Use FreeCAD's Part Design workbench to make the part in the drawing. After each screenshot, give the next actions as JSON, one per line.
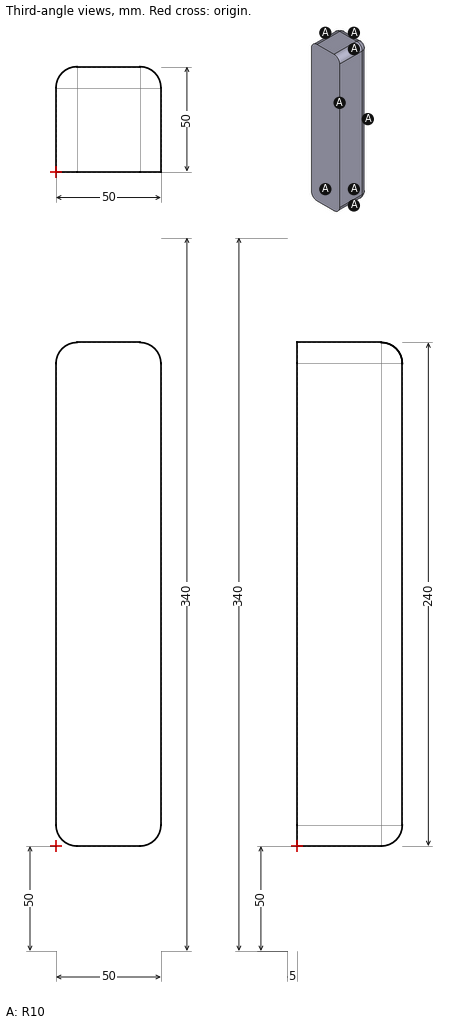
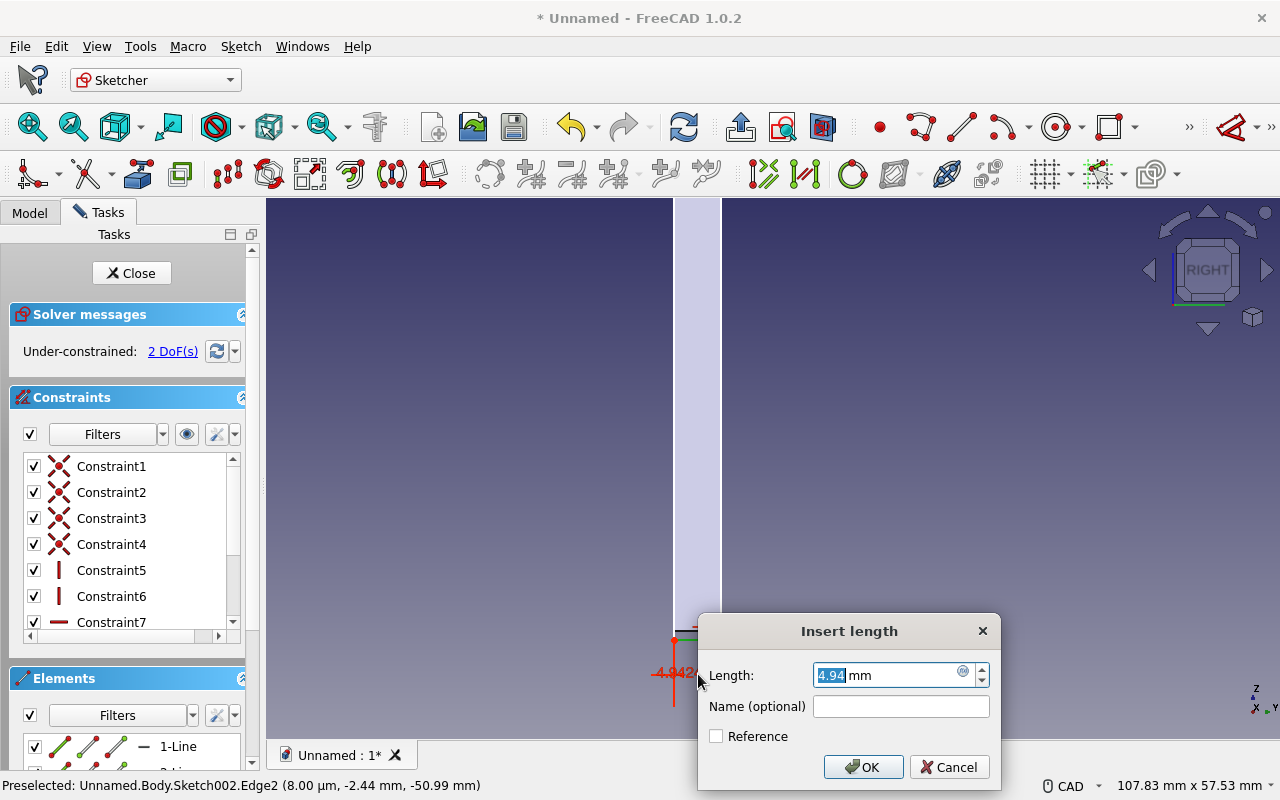
{"action": "type", "text": "5"}
{"action": "key", "text": "Return"}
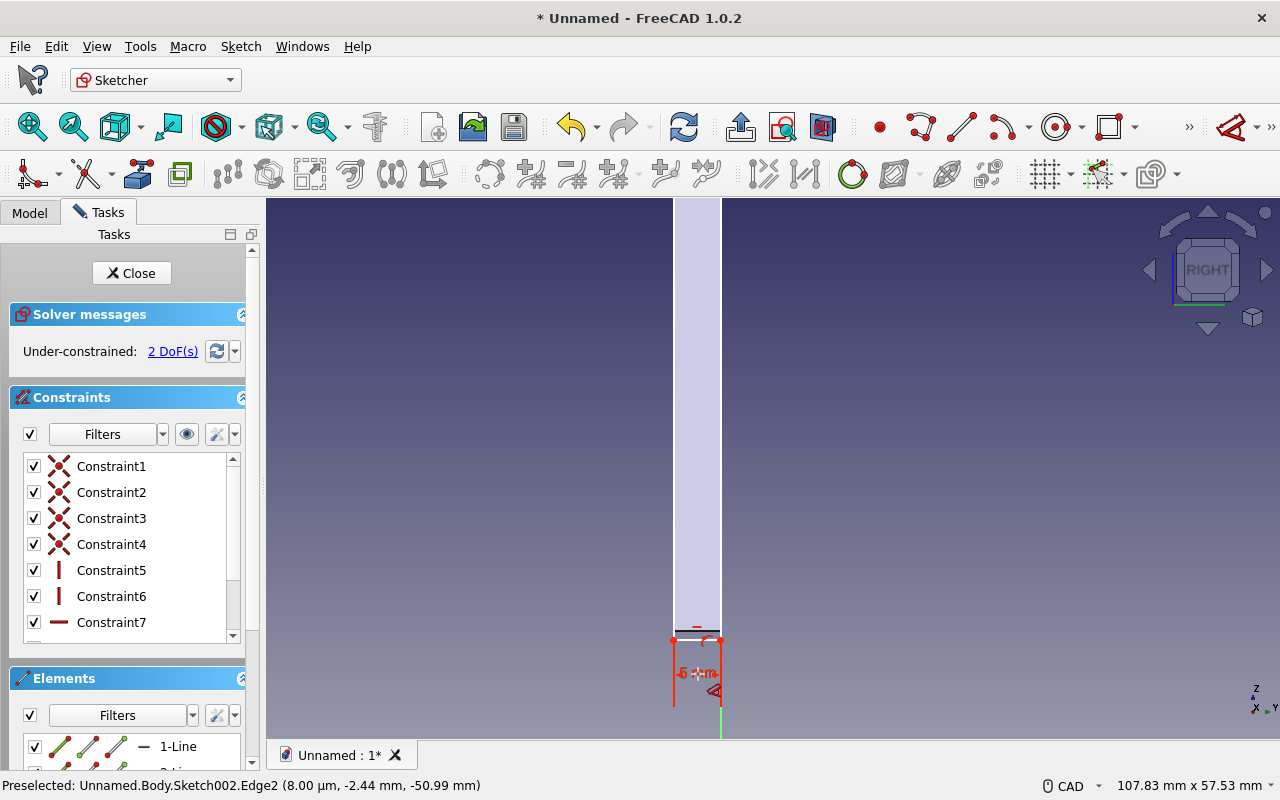
{"action": "scroll", "coordinate": [705, 647], "scroll_direction": "down", "scroll_amount": 11}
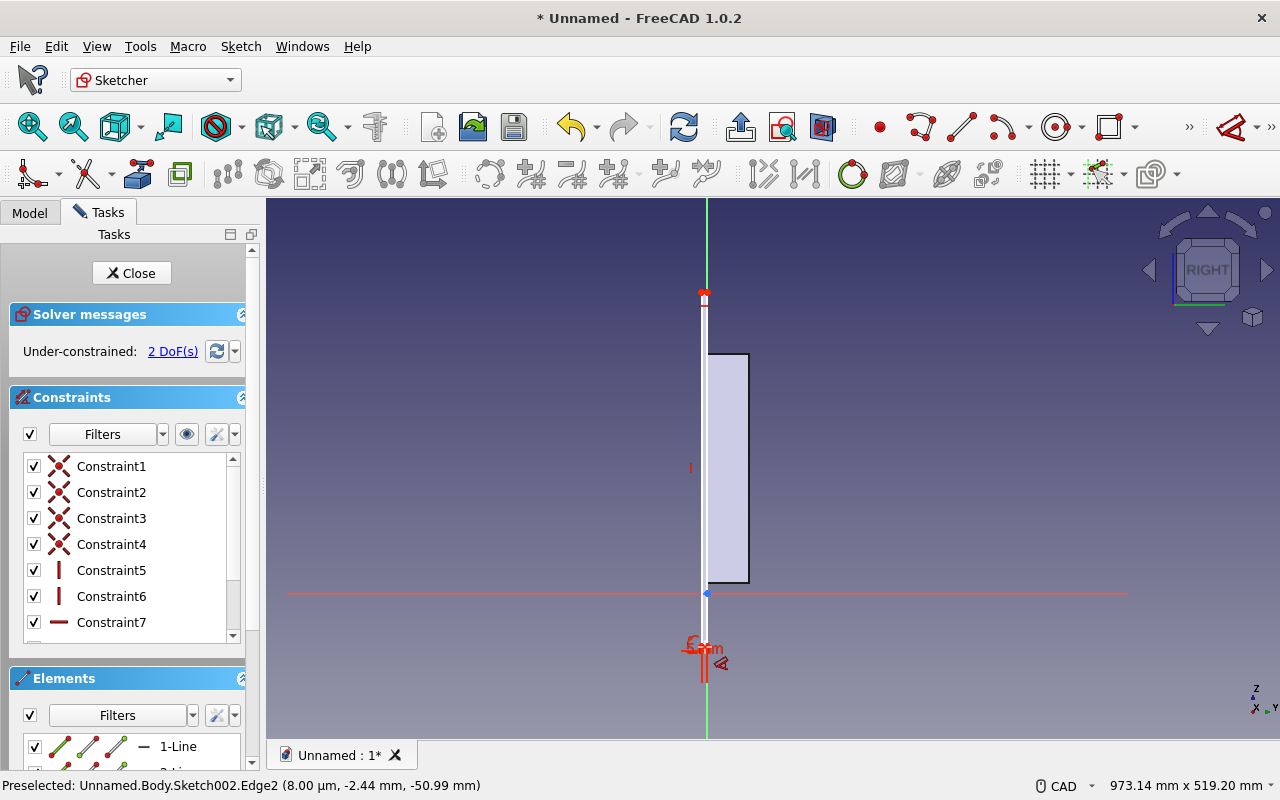
{"action": "scroll", "coordinate": [702, 399], "scroll_direction": "up", "scroll_amount": 5}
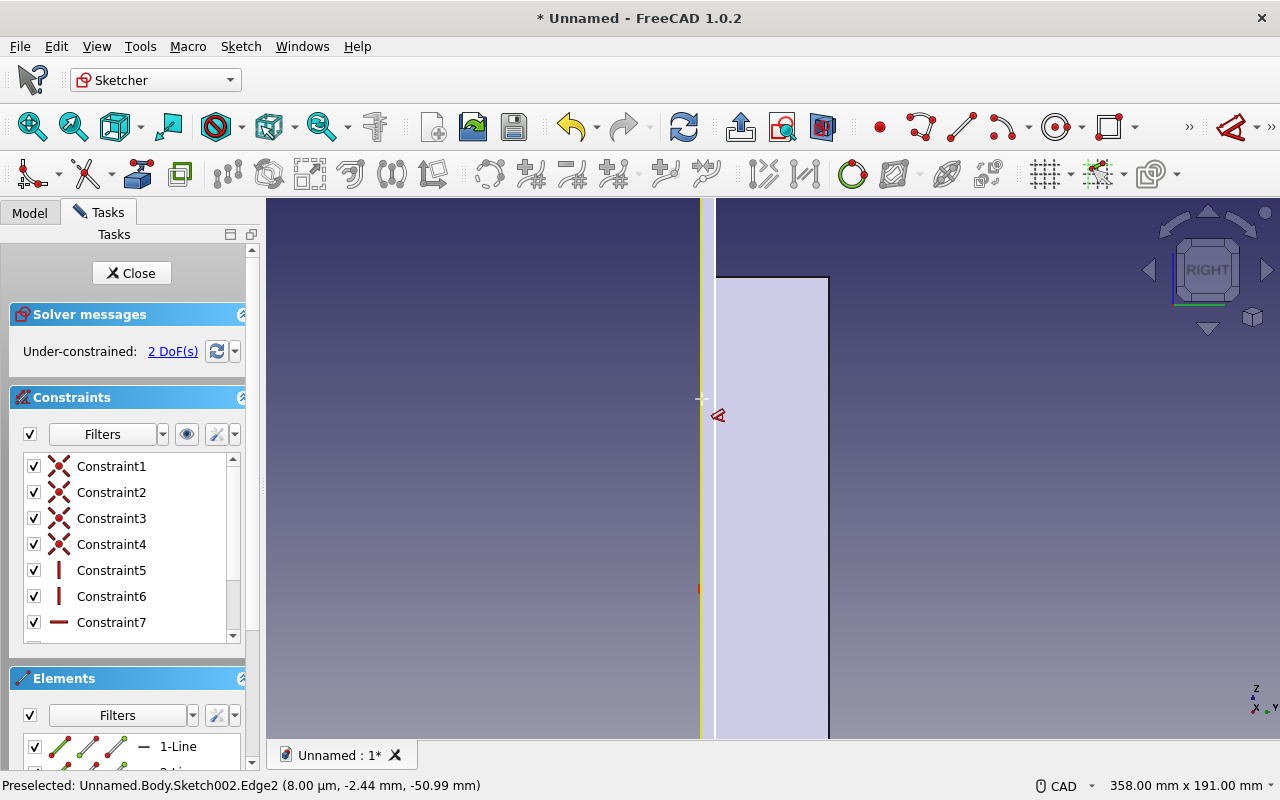
{"action": "left_click", "coordinate": [701, 397]}
{"action": "left_click", "coordinate": [667, 468]}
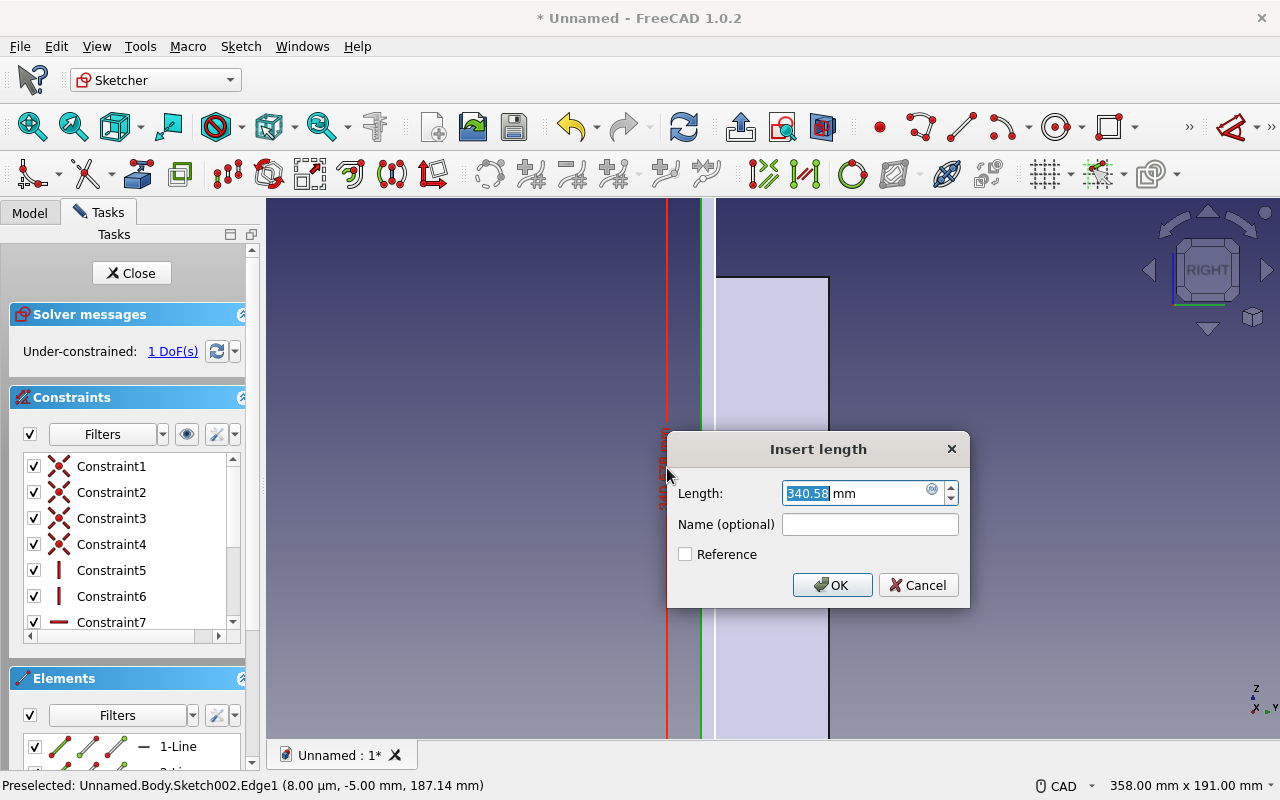
{"action": "type", "text": "340"}
{"action": "key", "text": "Return"}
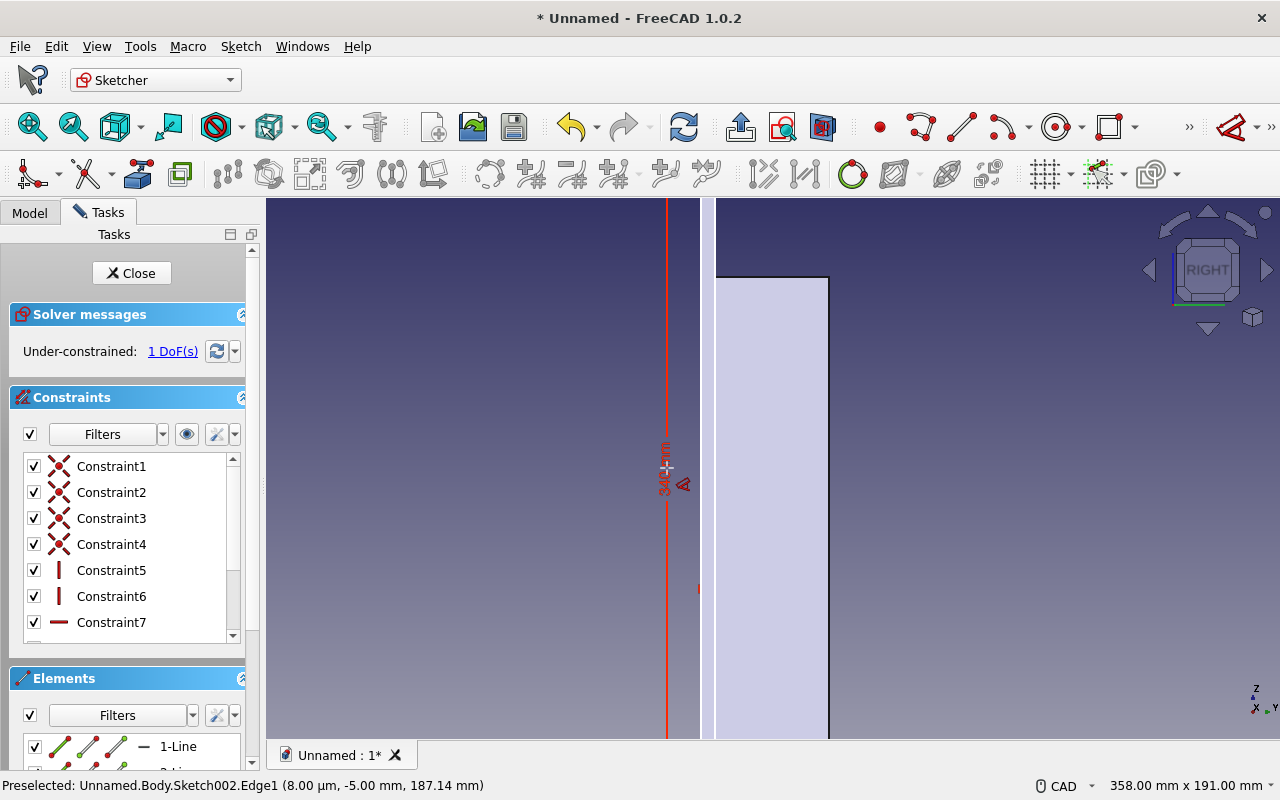
{"action": "scroll", "coordinate": [702, 399], "scroll_direction": "down", "scroll_amount": 5}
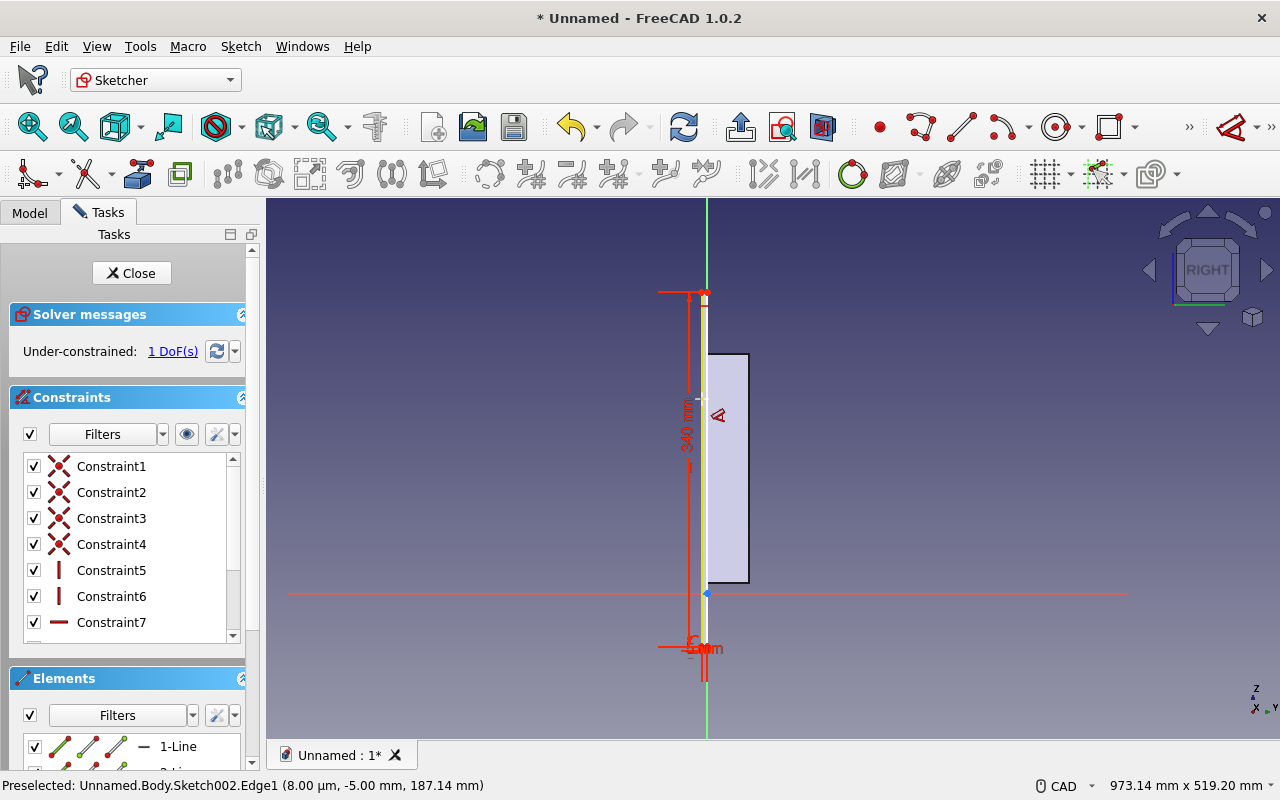
{"action": "scroll", "coordinate": [702, 647], "scroll_direction": "up", "scroll_amount": 5}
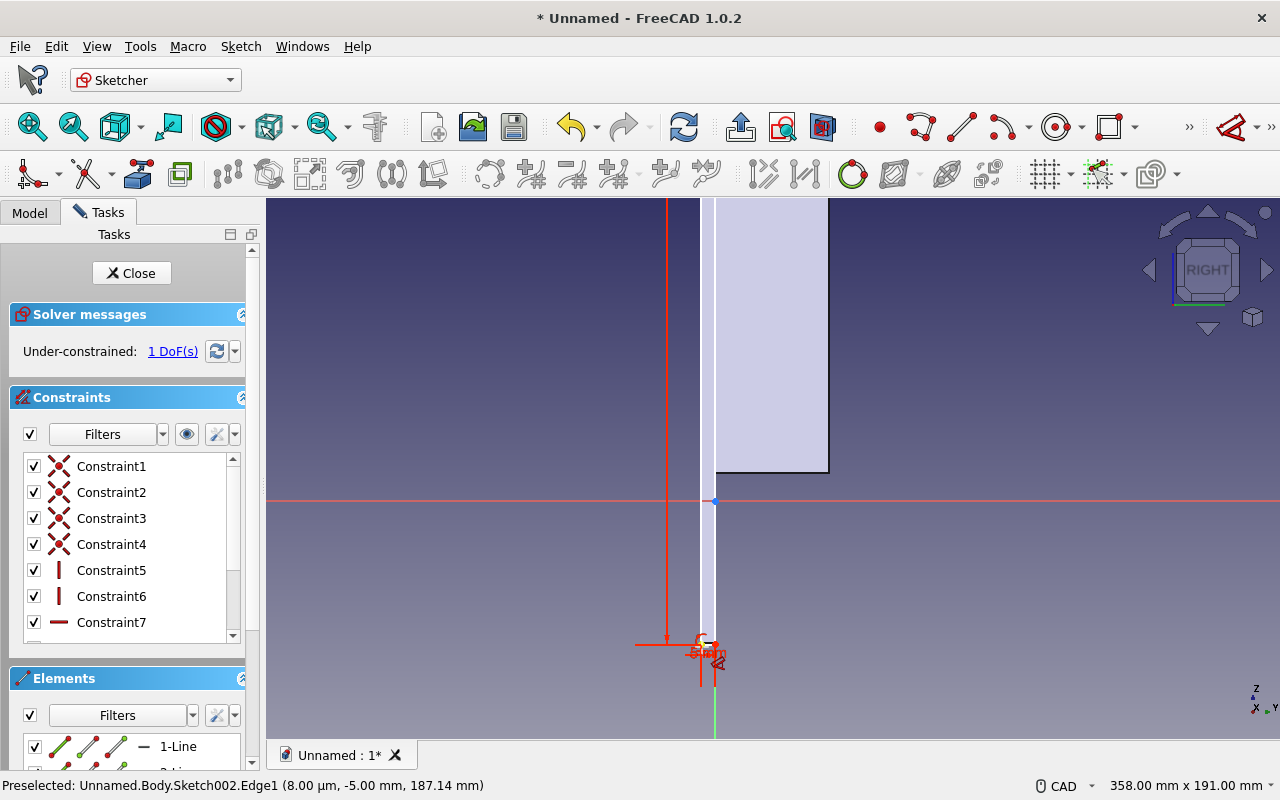
{"action": "left_click", "coordinate": [701, 645]}
{"action": "left_click", "coordinate": [667, 573]}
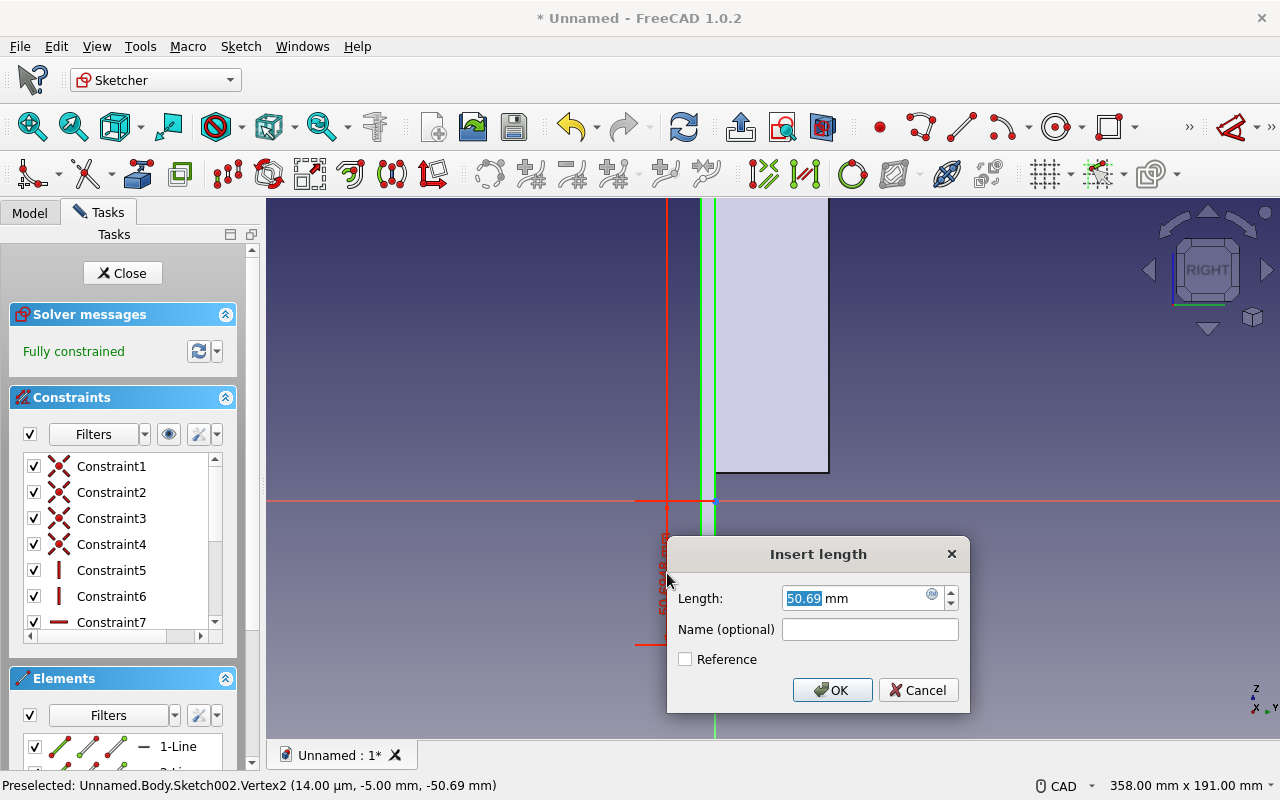
{"action": "type", "text": "50"}
{"action": "key", "text": "Return"}
{"action": "key", "text": "Escape"}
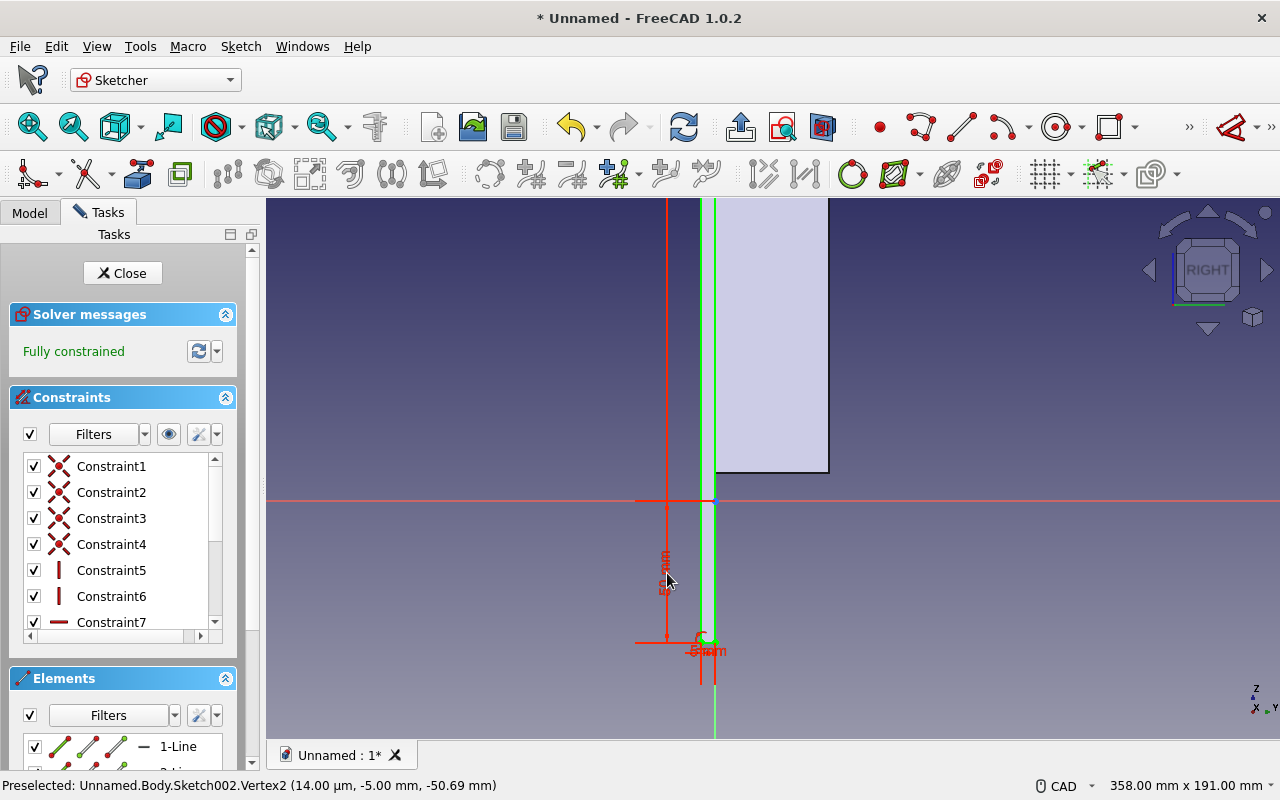
{"action": "left_click", "coordinate": [123, 273]}